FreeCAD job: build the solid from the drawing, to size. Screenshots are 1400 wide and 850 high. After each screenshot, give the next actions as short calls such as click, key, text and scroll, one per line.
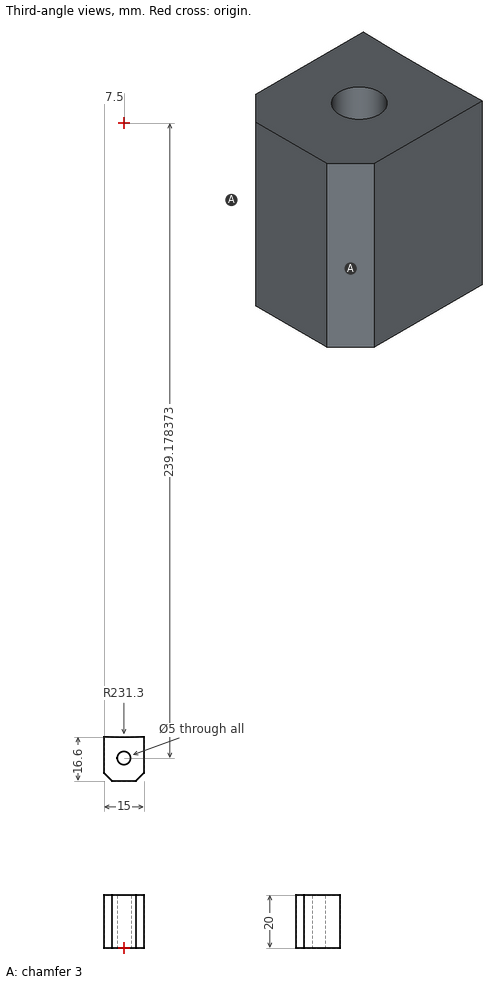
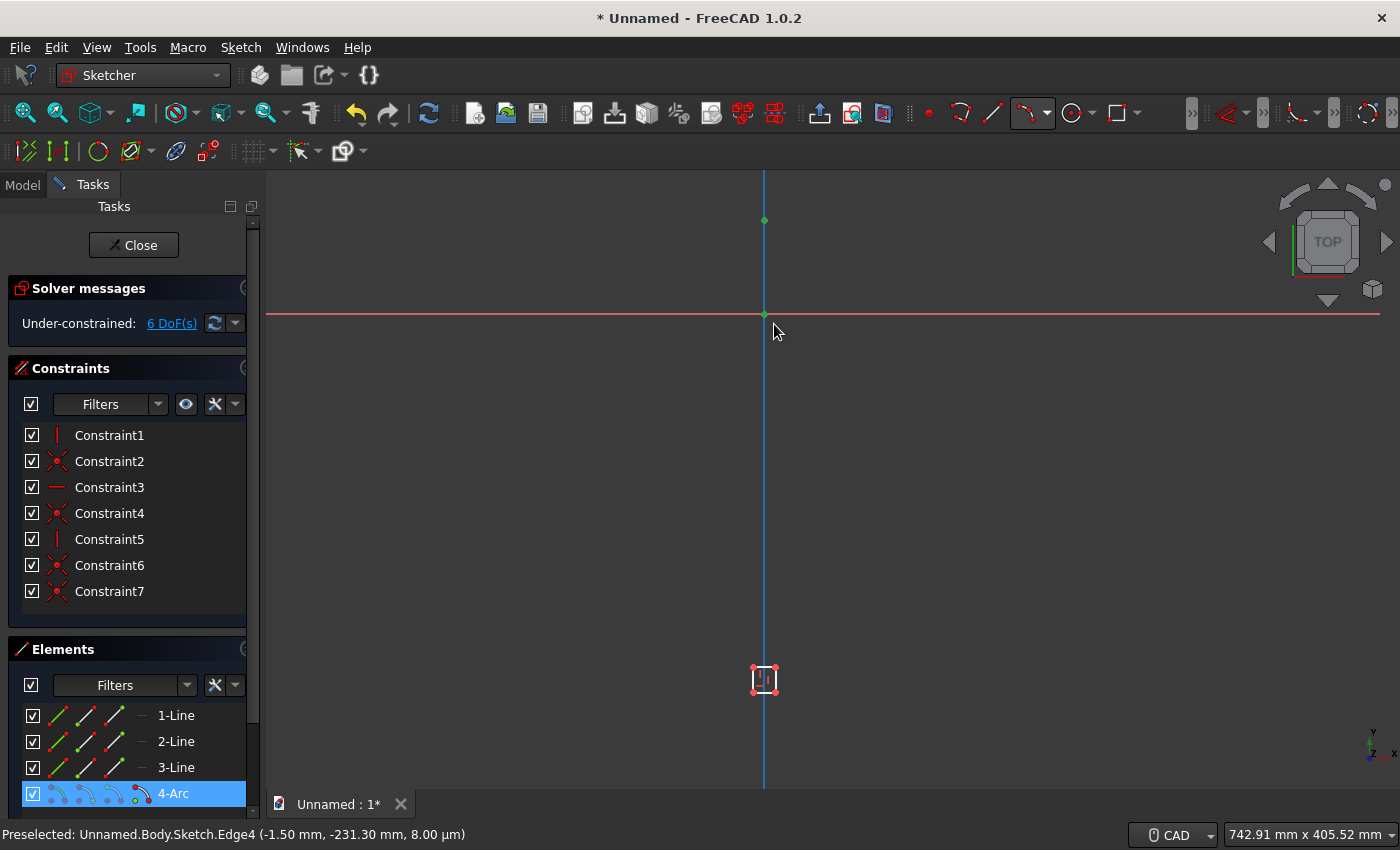
key(c)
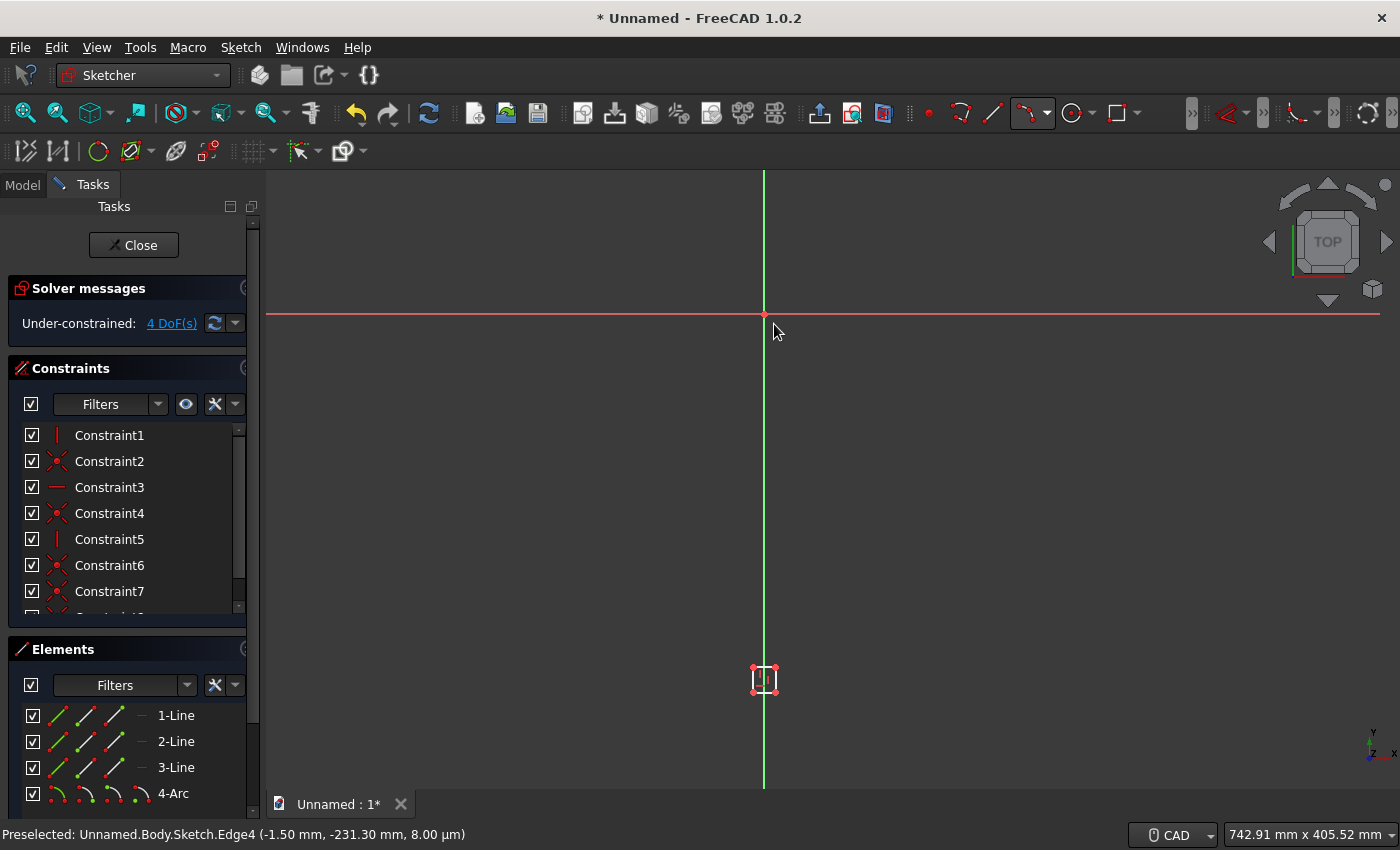
click(1226, 114)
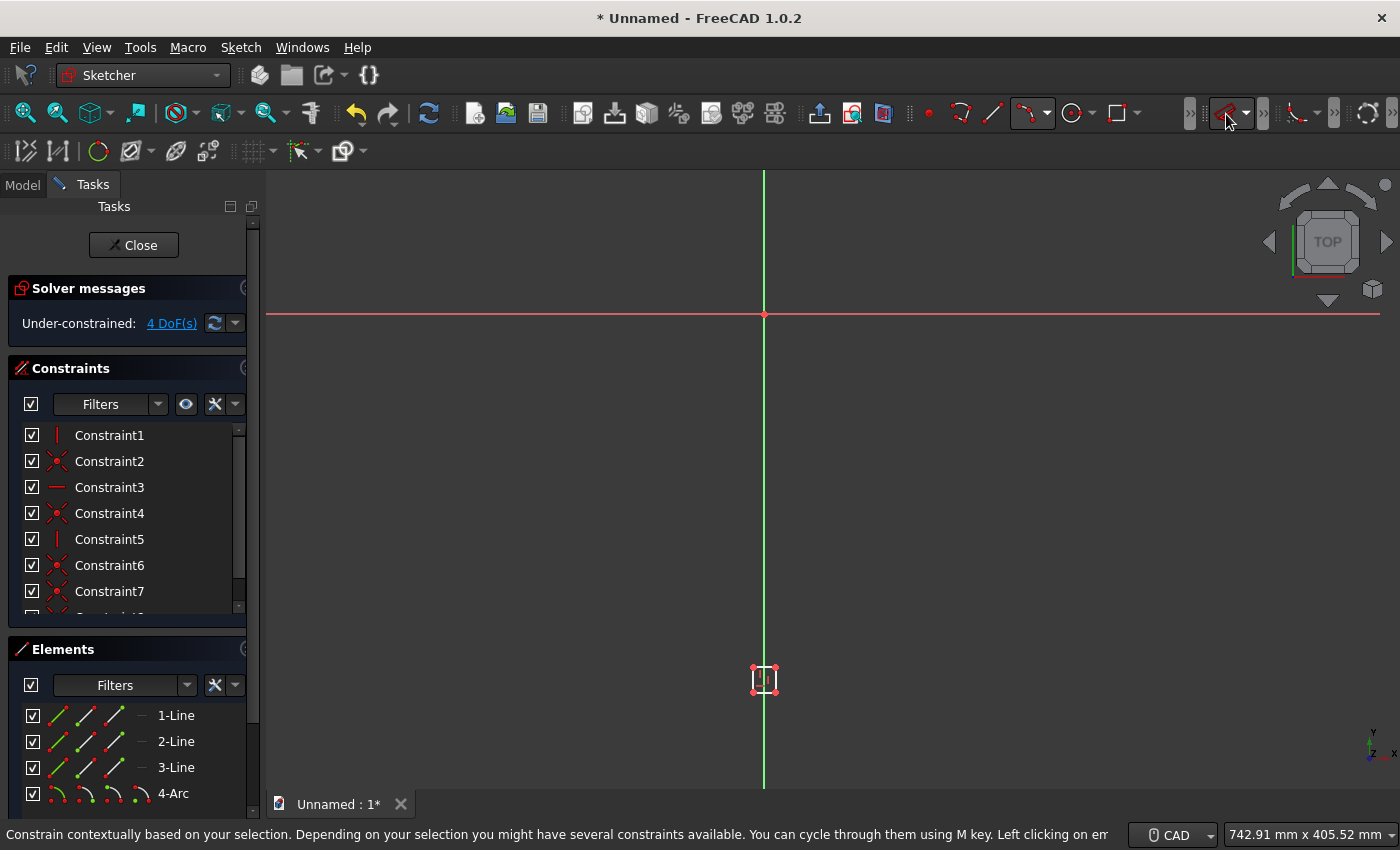
click(764, 667)
click(580, 652)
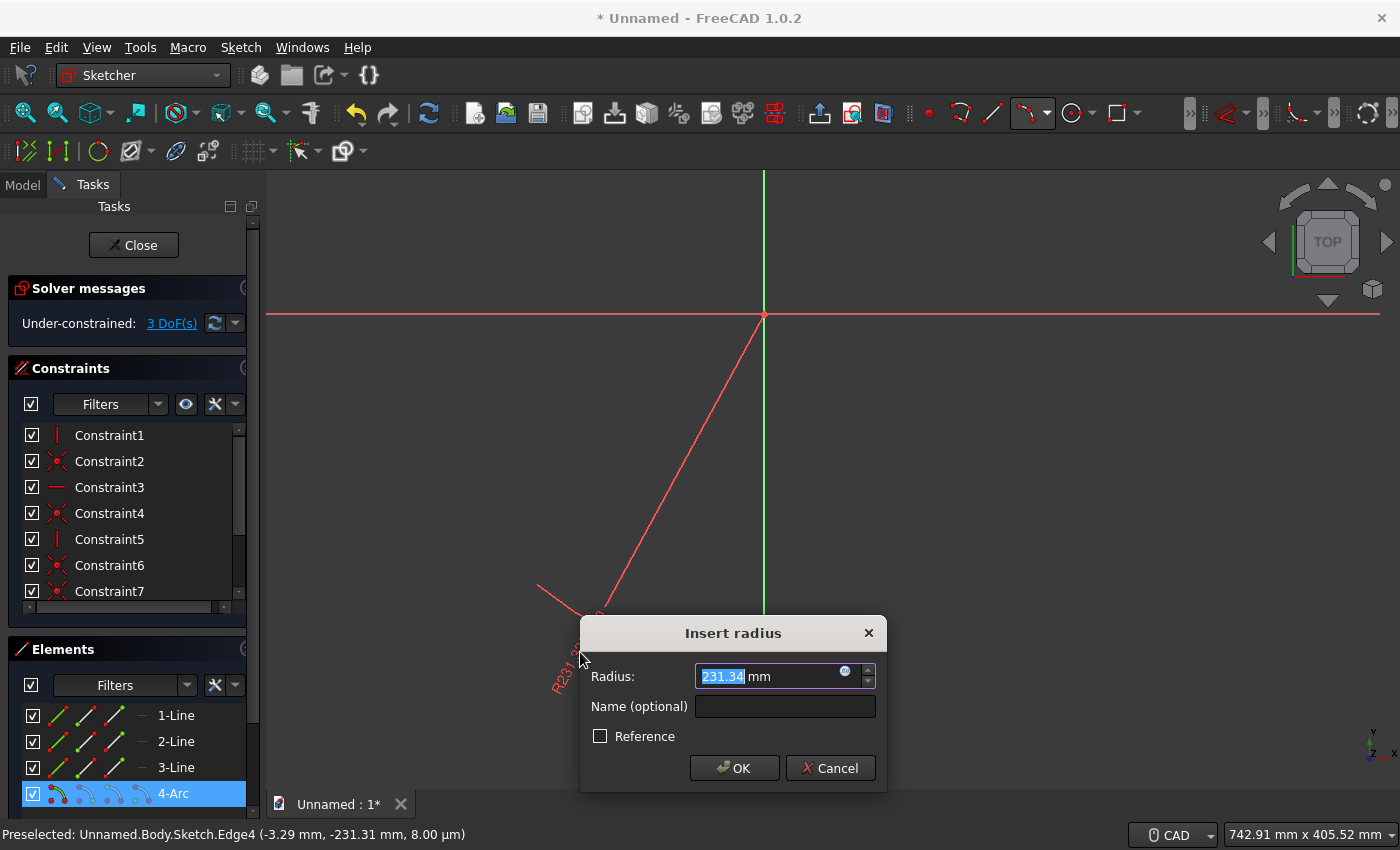
text(231.3)
key(Return)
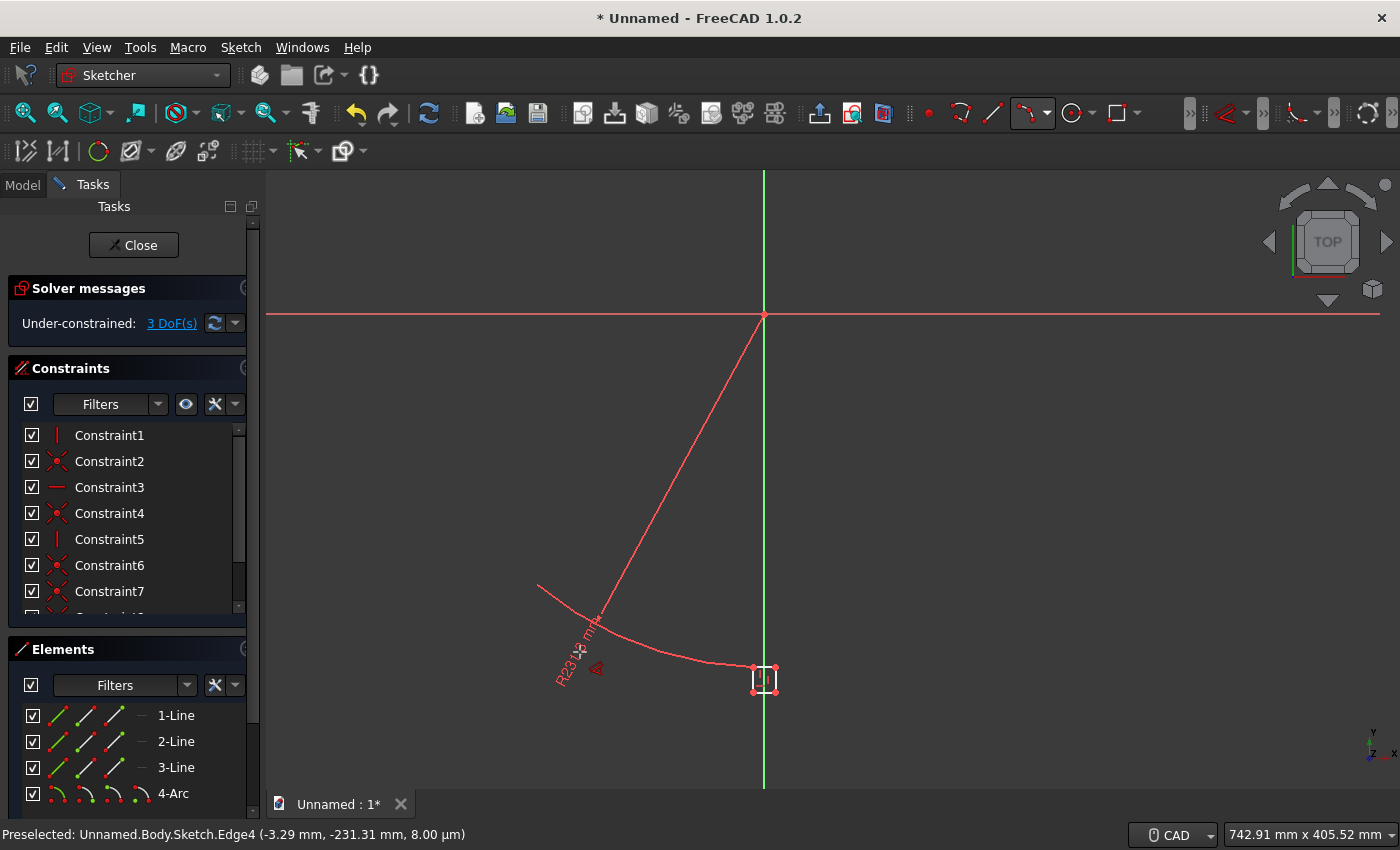
scroll(762, 693, up, 3)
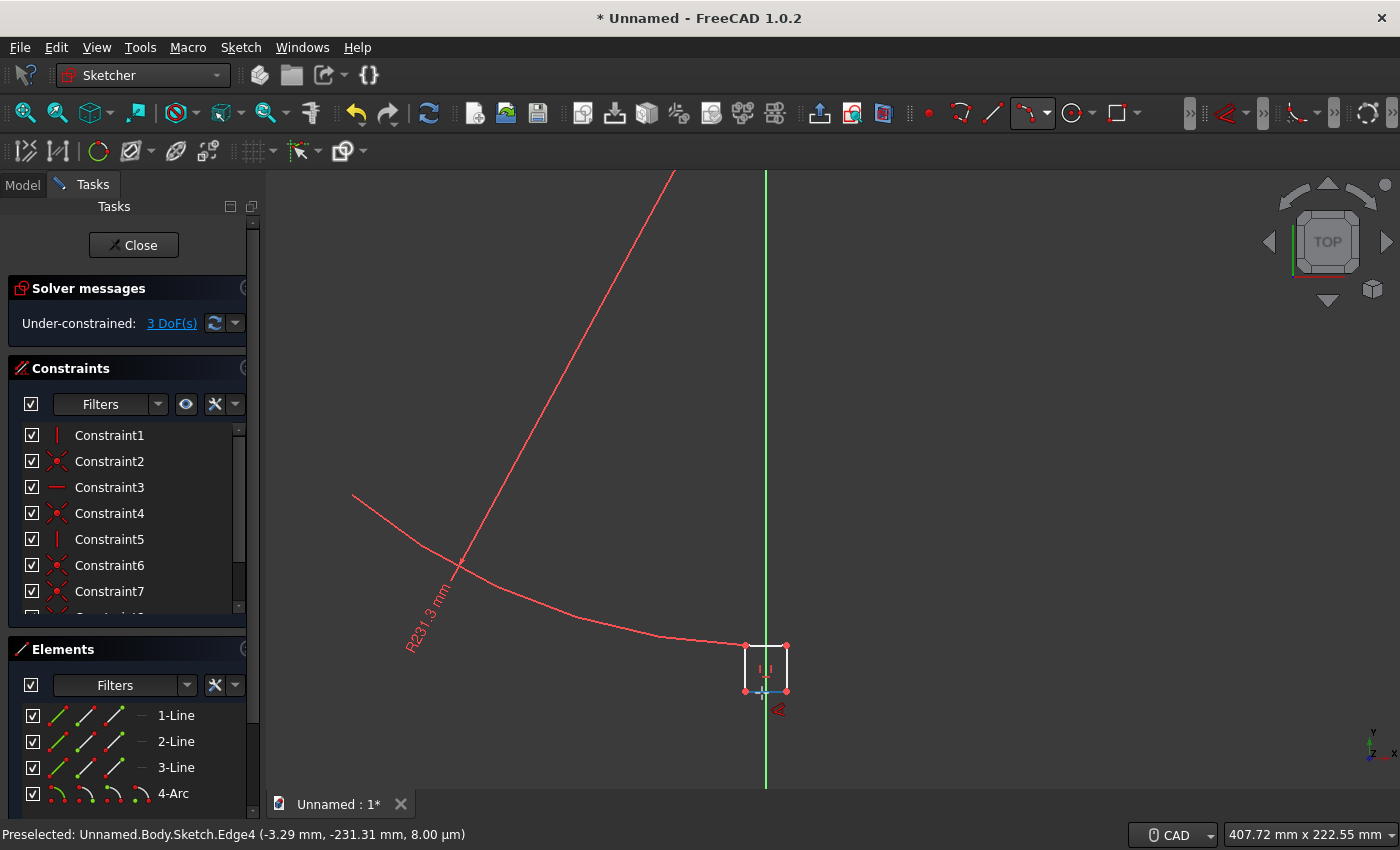
click(762, 692)
click(752, 726)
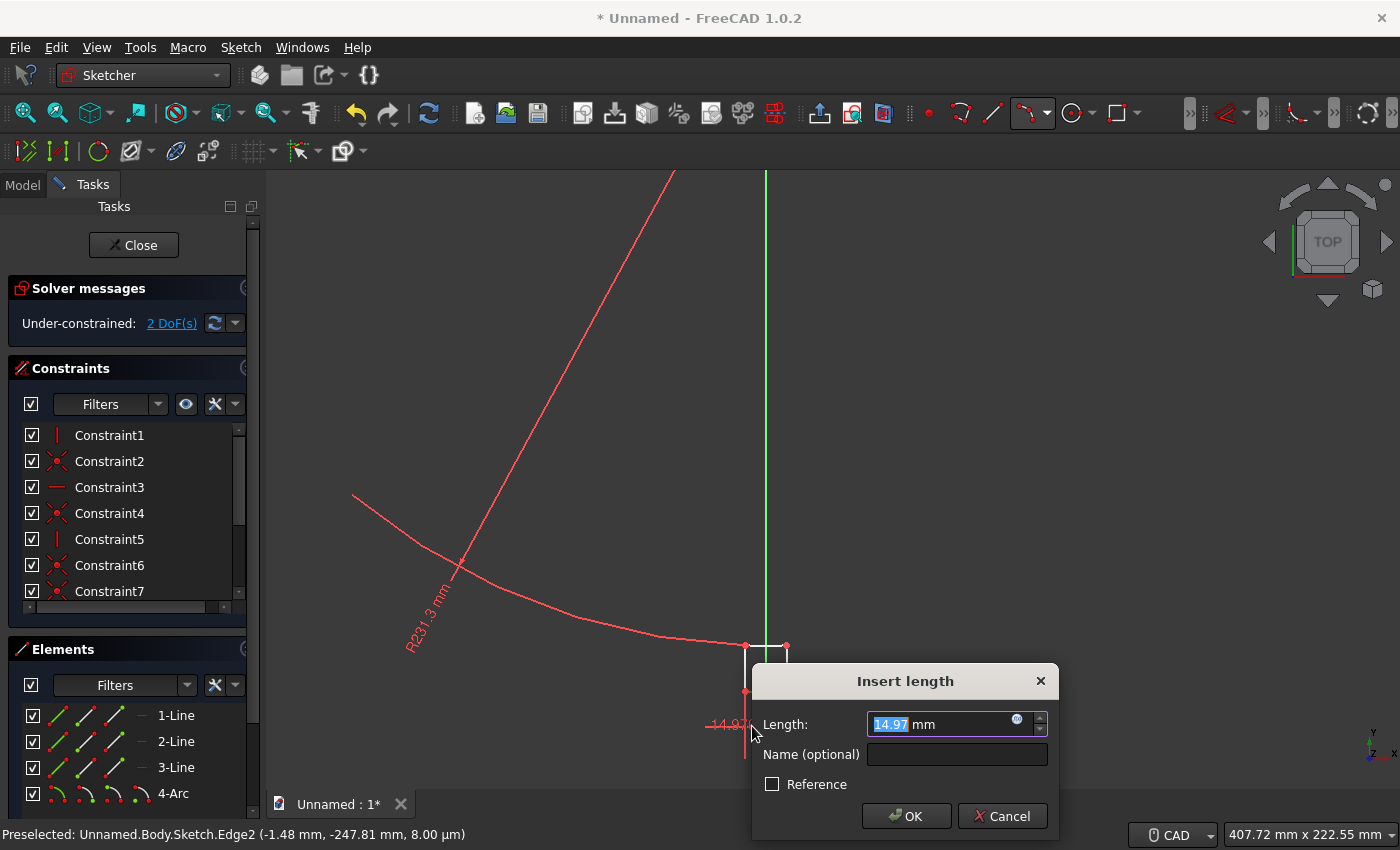
text(15)
key(Return)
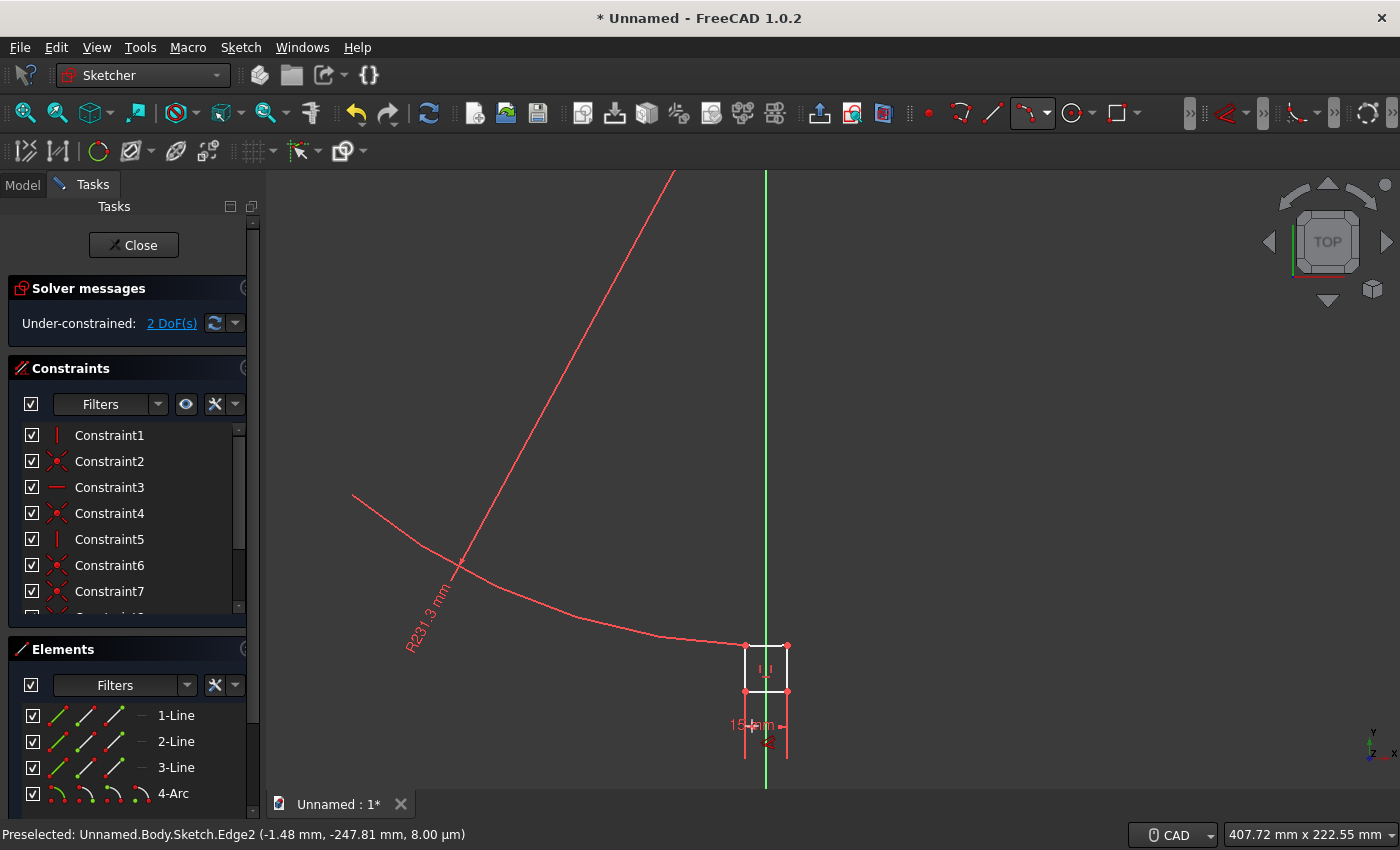
click(745, 659)
click(711, 668)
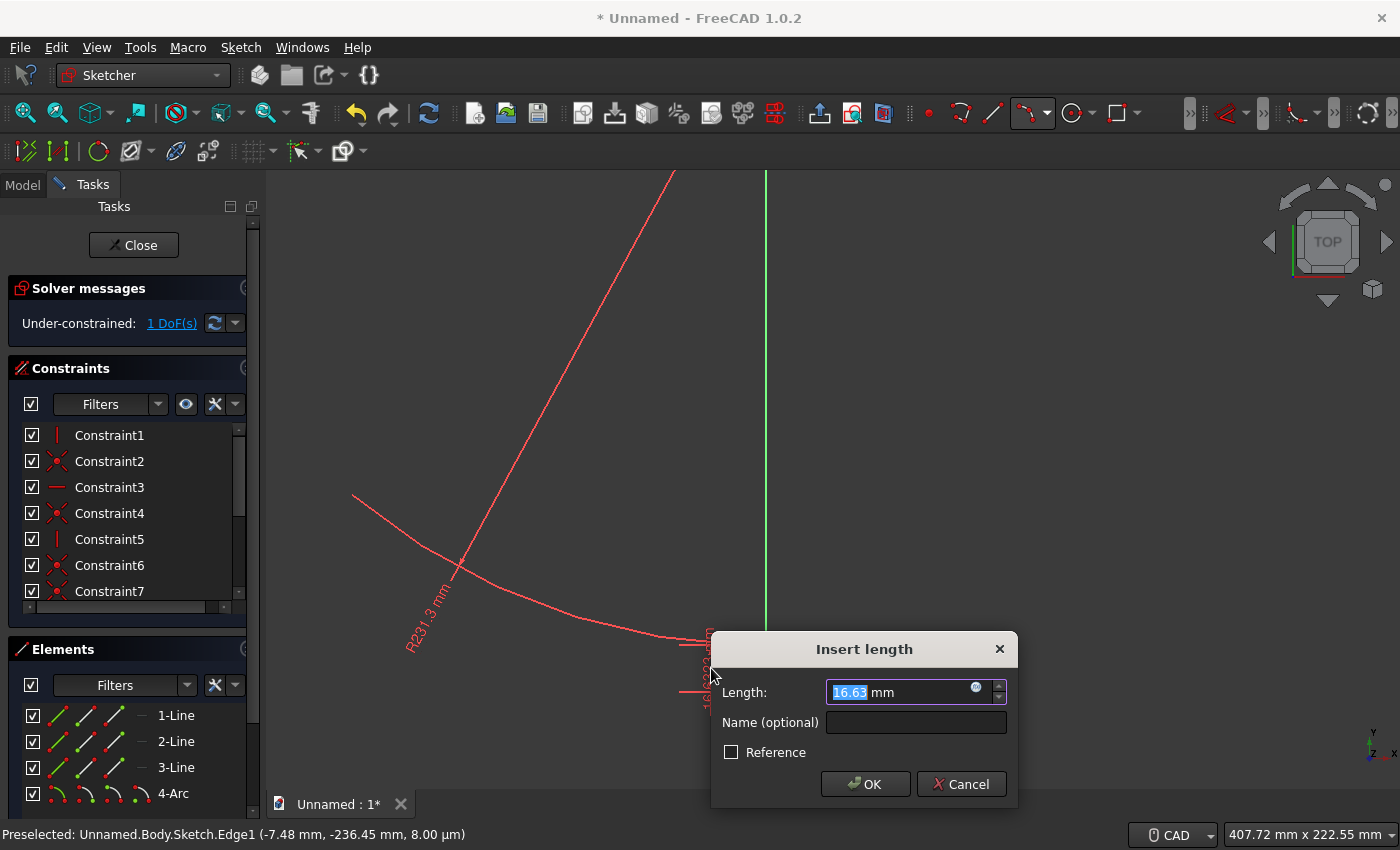
text(16.6)
key(Return)